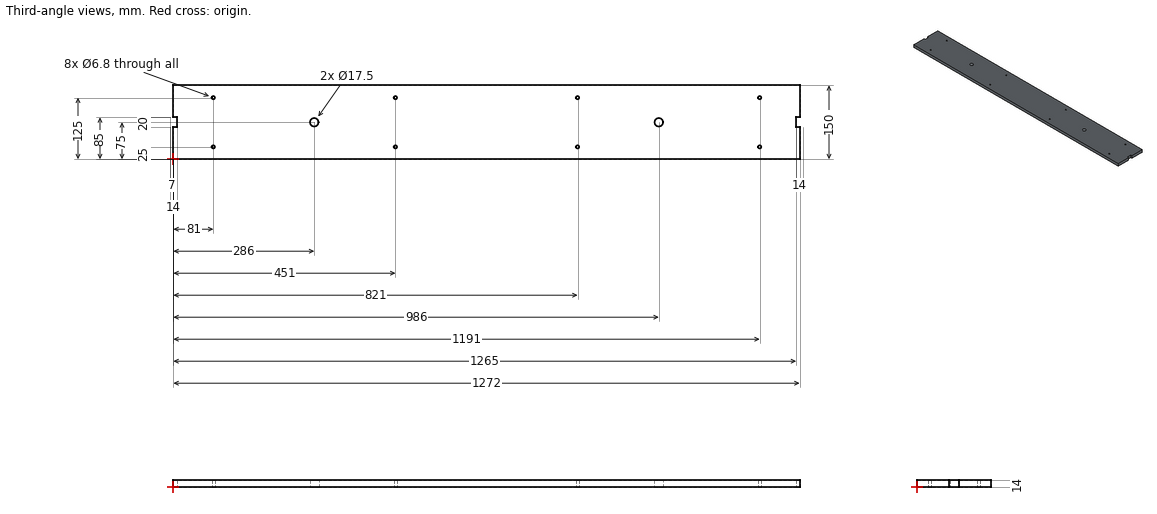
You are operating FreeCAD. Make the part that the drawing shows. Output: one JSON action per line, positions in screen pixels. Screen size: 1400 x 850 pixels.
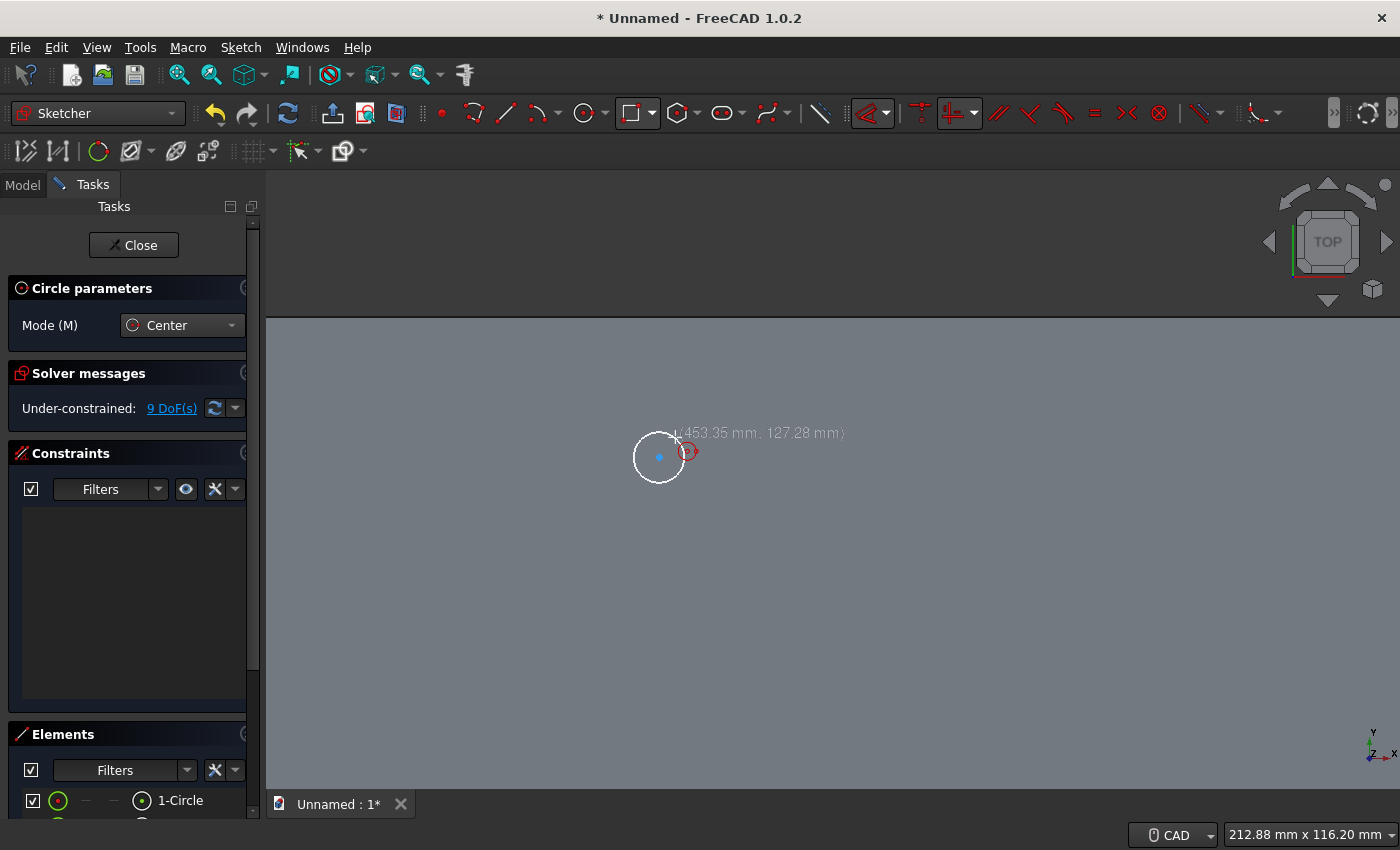
{"action": "scroll", "coordinate": [680, 443], "scroll_direction": "down", "scroll_amount": 11}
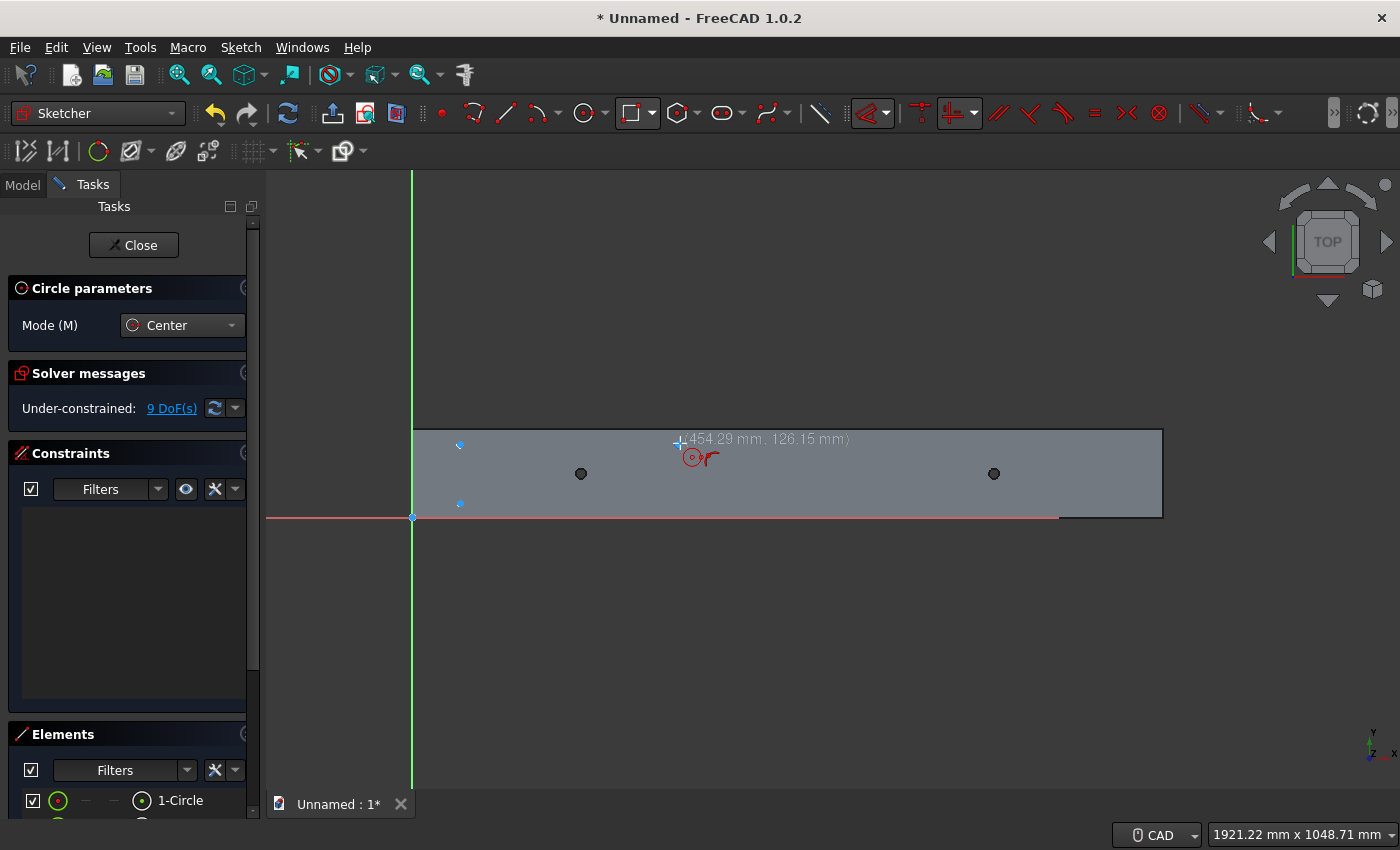
{"action": "scroll", "coordinate": [678, 503], "scroll_direction": "up", "scroll_amount": 13}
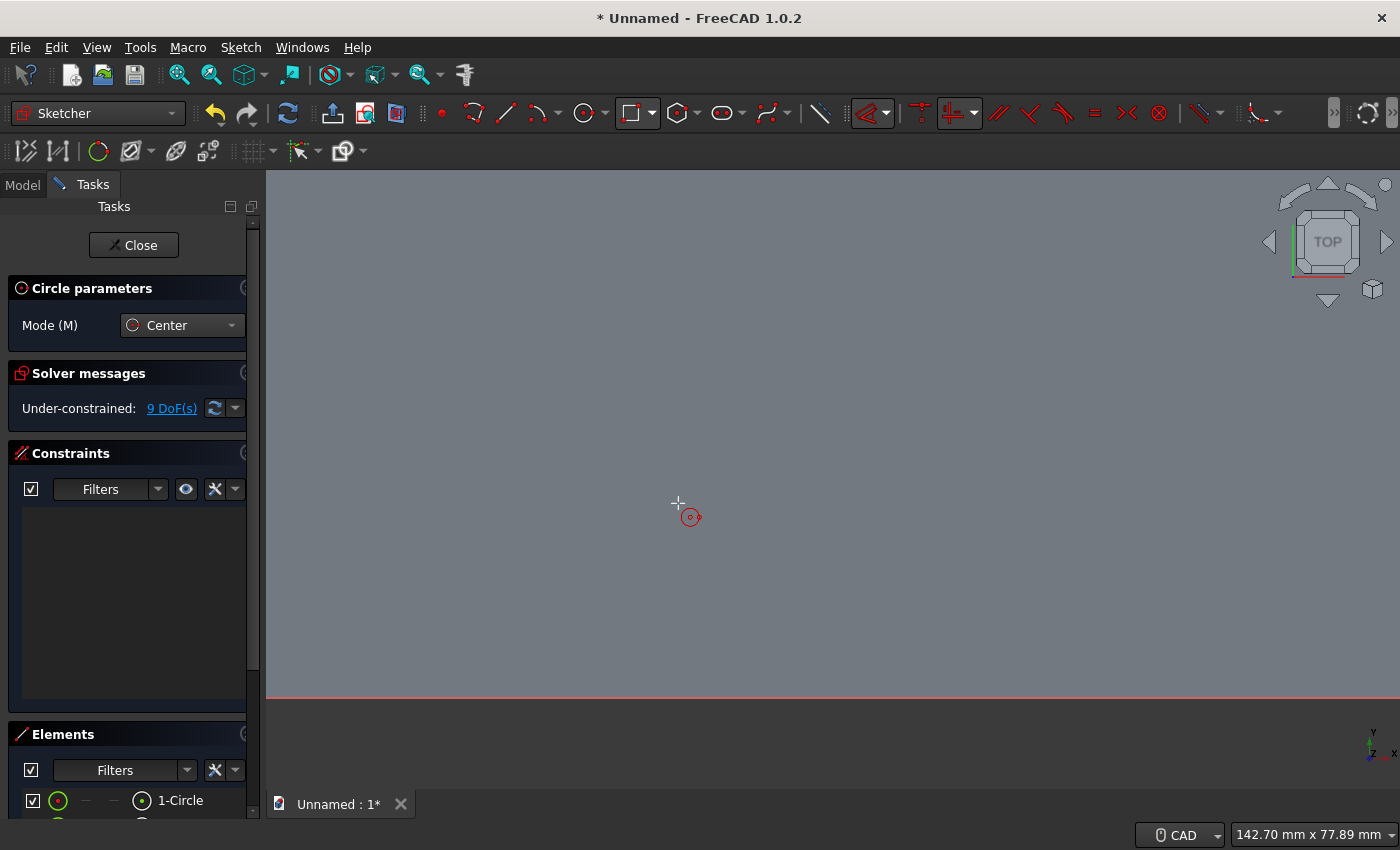
{"action": "scroll", "coordinate": [678, 503], "scroll_direction": "down", "scroll_amount": 13}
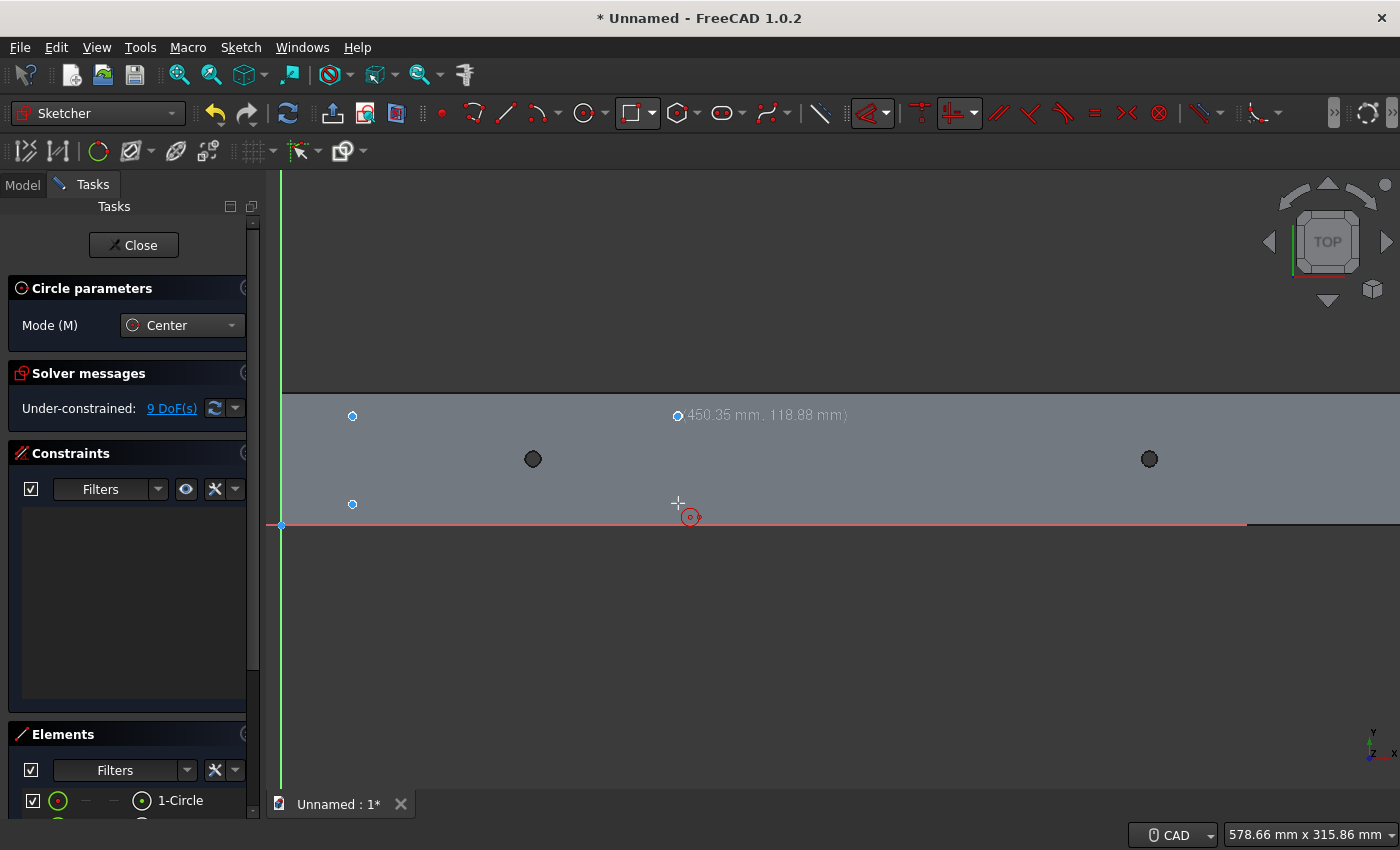
{"action": "left_click", "coordinate": [678, 503]}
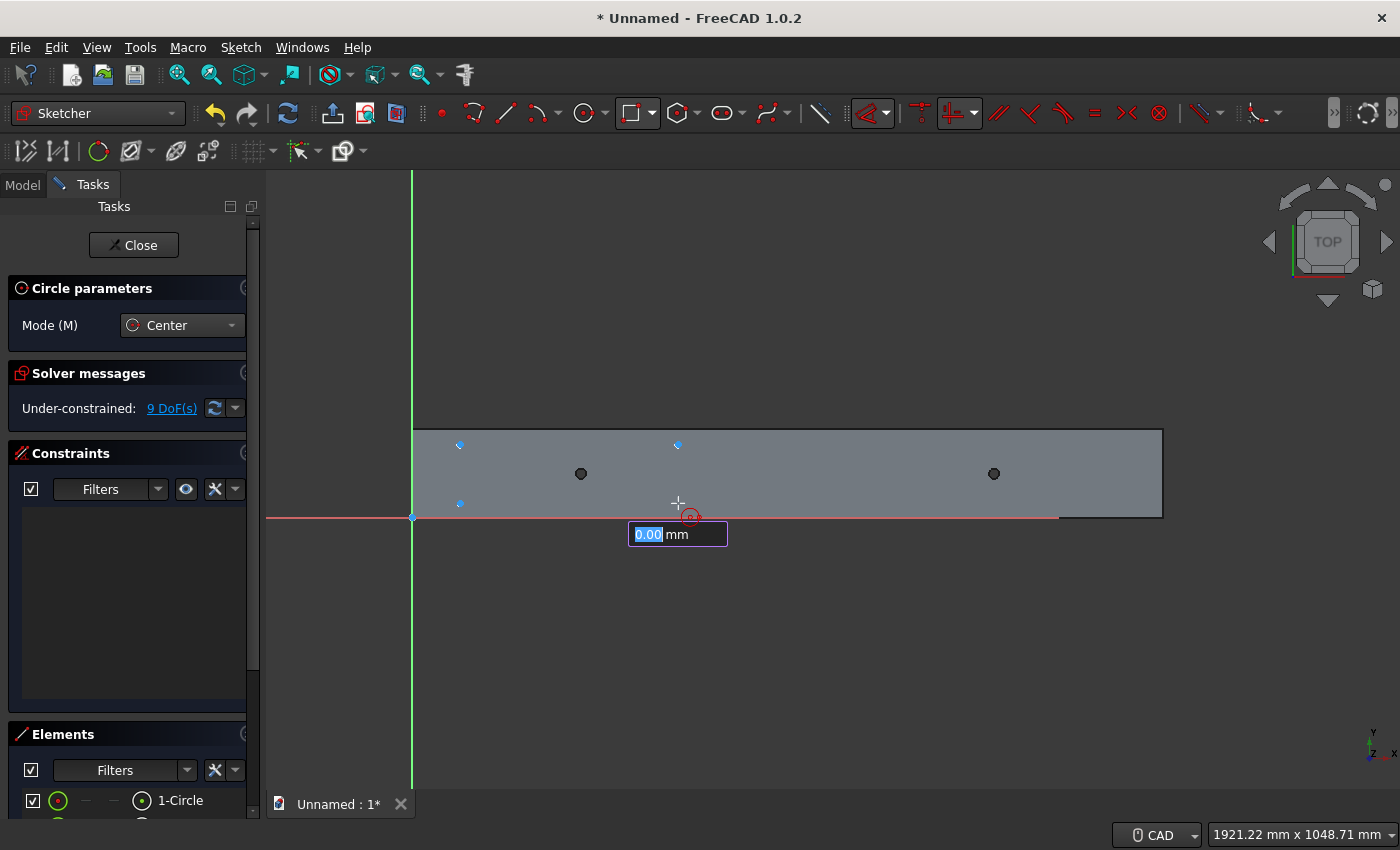
{"action": "scroll", "coordinate": [680, 502], "scroll_direction": "up", "scroll_amount": 11}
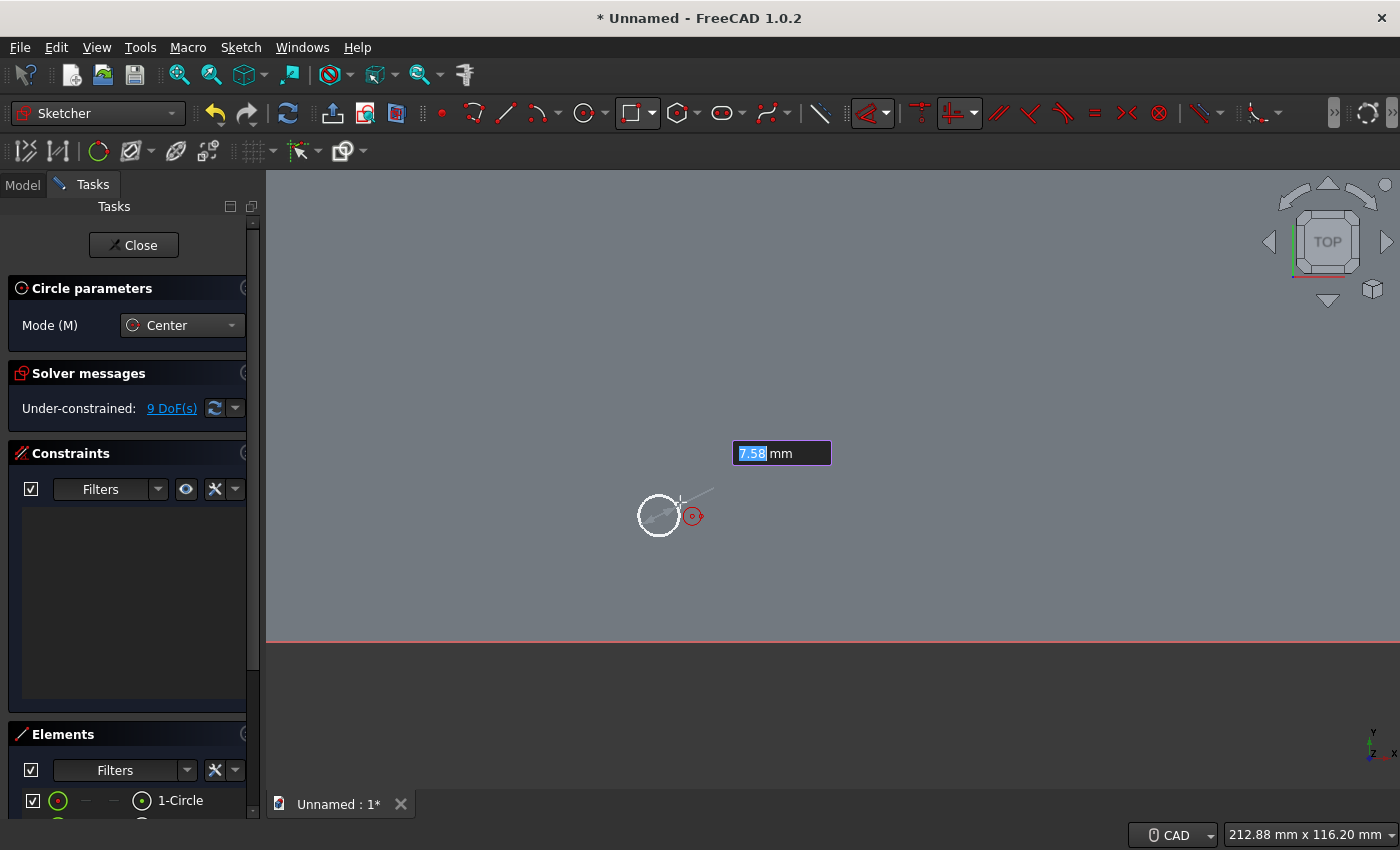
{"action": "left_click", "coordinate": [675, 496]}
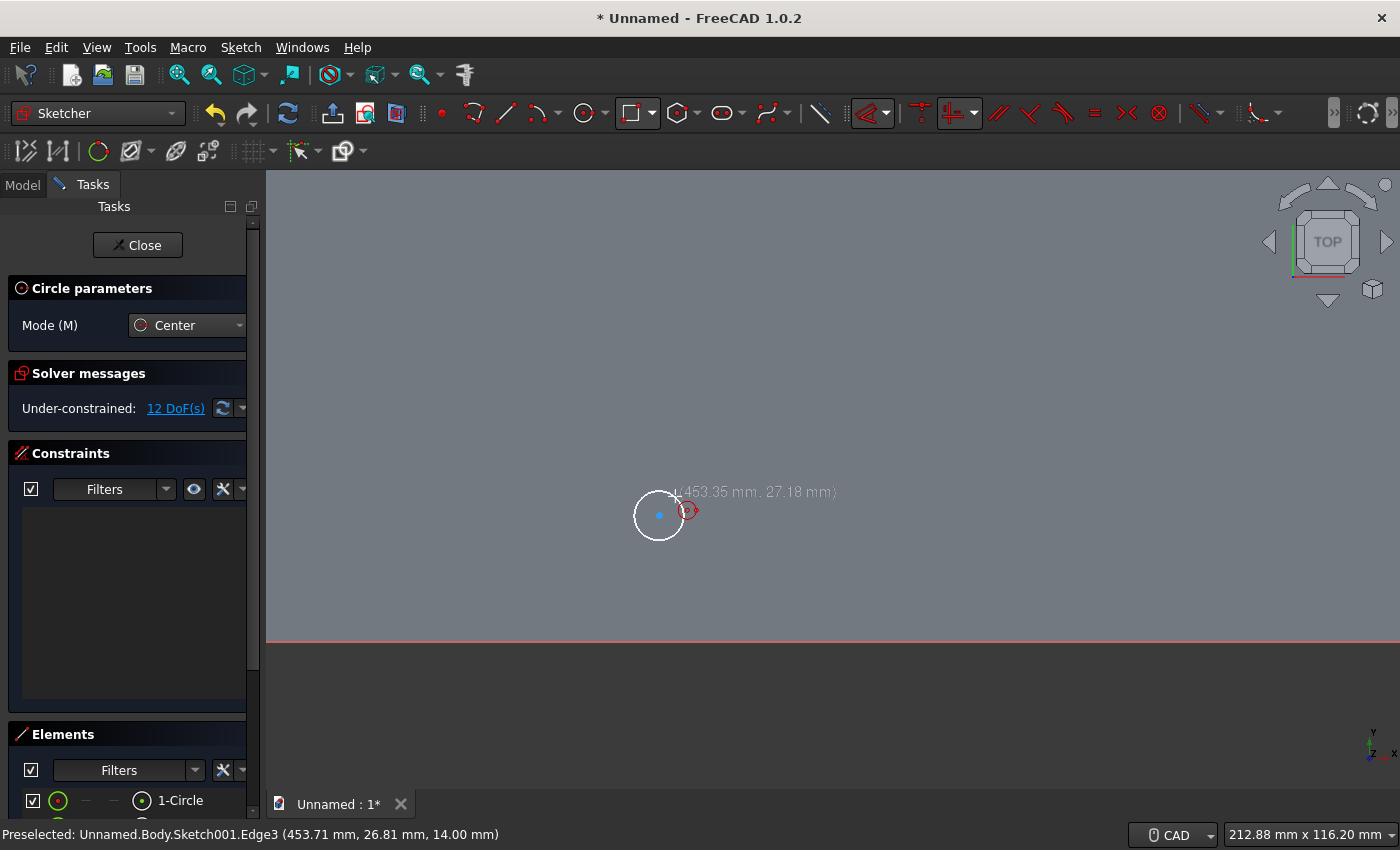
{"action": "scroll", "coordinate": [680, 502], "scroll_direction": "down", "scroll_amount": 11}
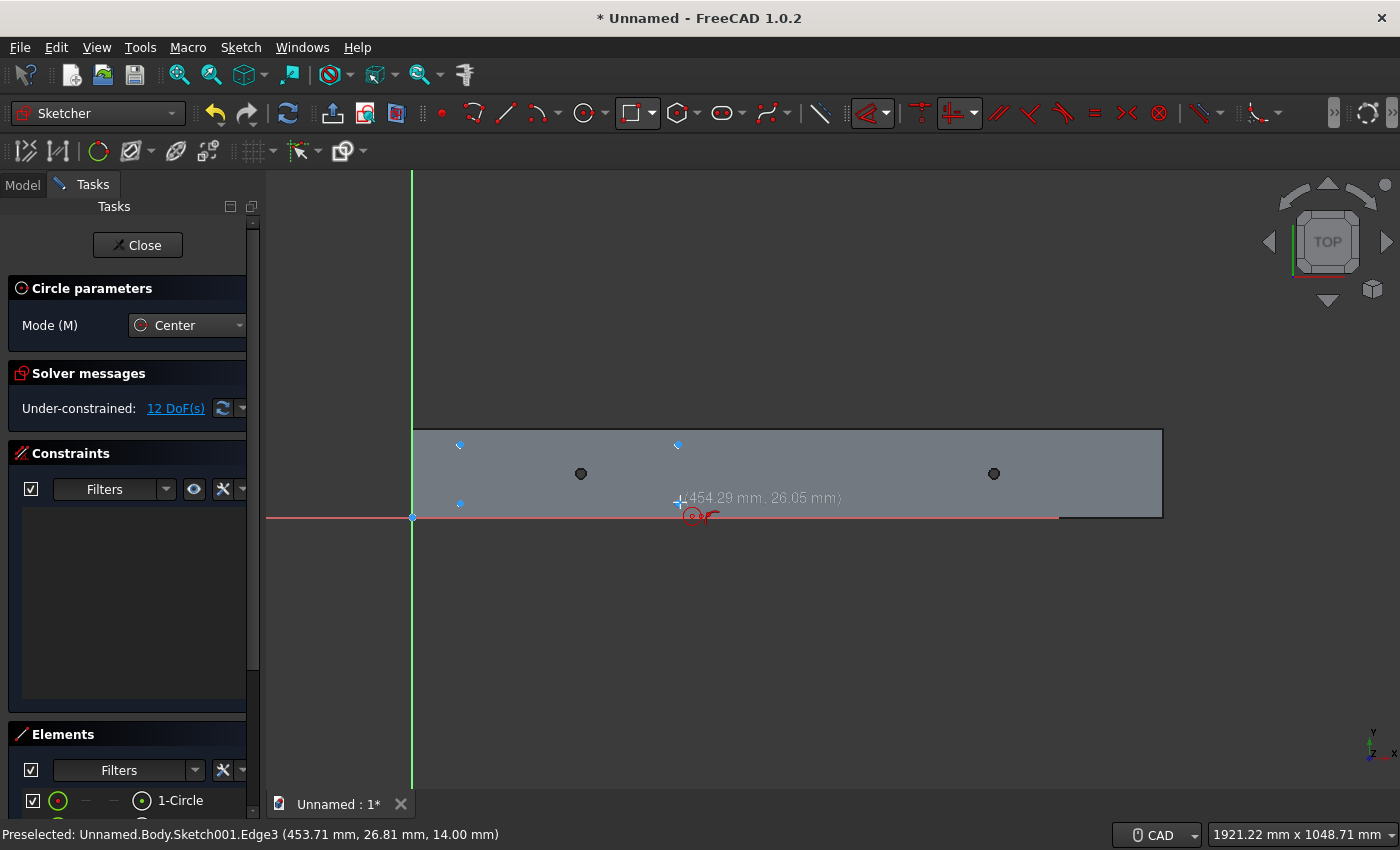
{"action": "scroll", "coordinate": [897, 444], "scroll_direction": "up", "scroll_amount": 13}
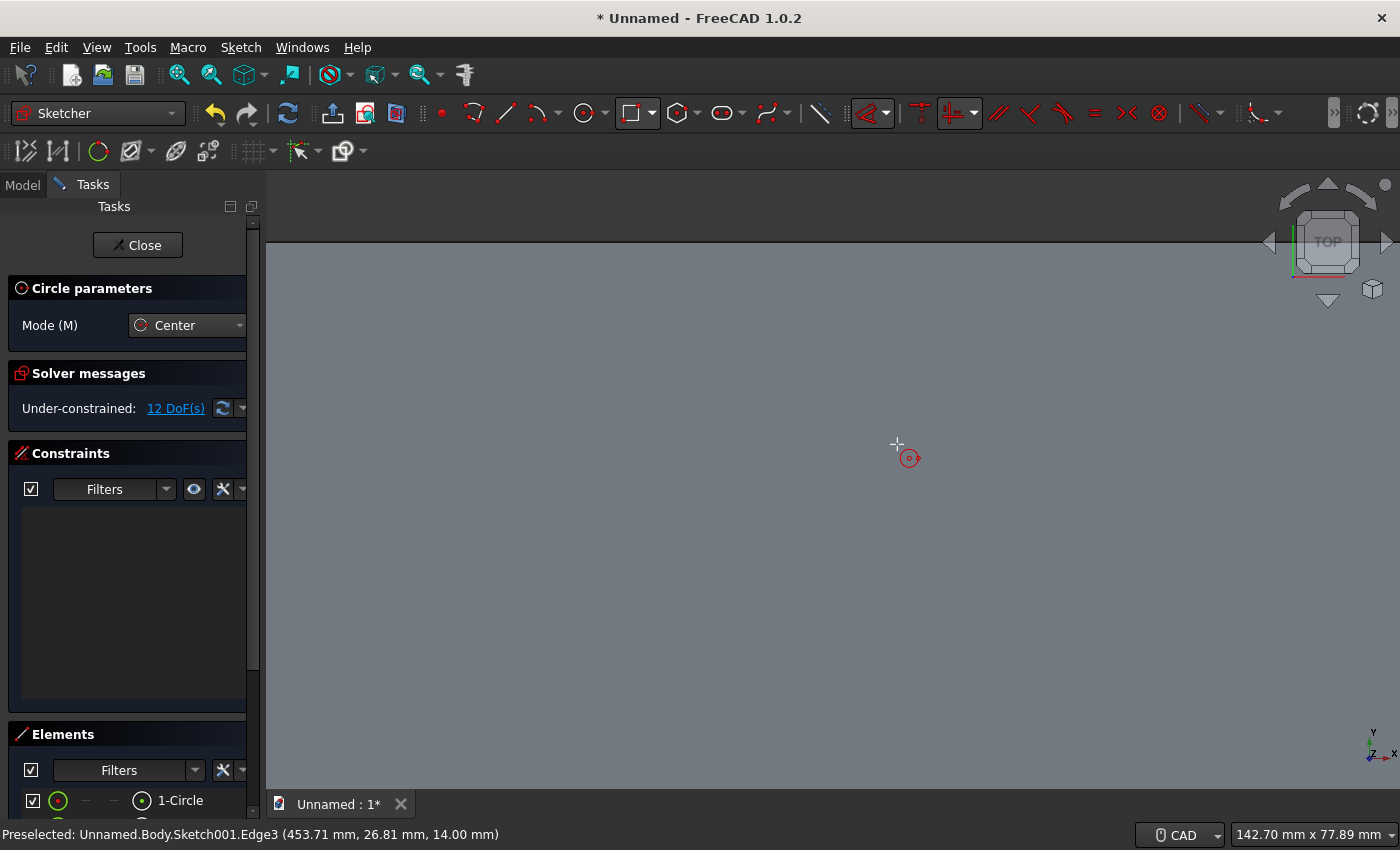
{"action": "scroll", "coordinate": [897, 444], "scroll_direction": "down", "scroll_amount": 13}